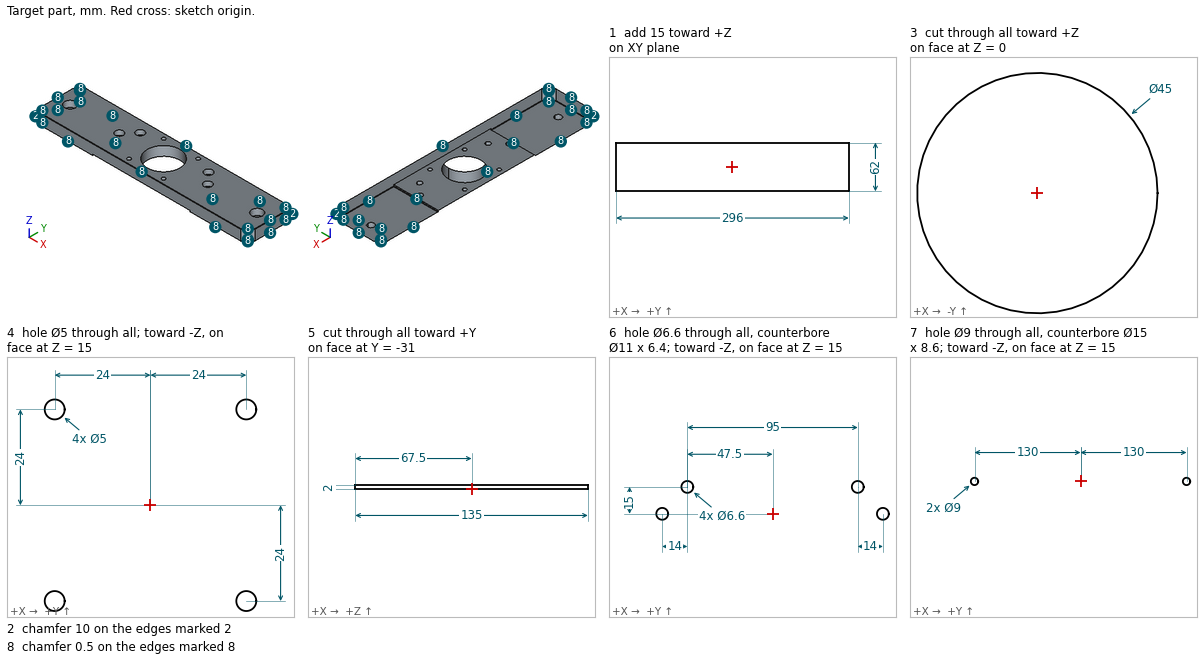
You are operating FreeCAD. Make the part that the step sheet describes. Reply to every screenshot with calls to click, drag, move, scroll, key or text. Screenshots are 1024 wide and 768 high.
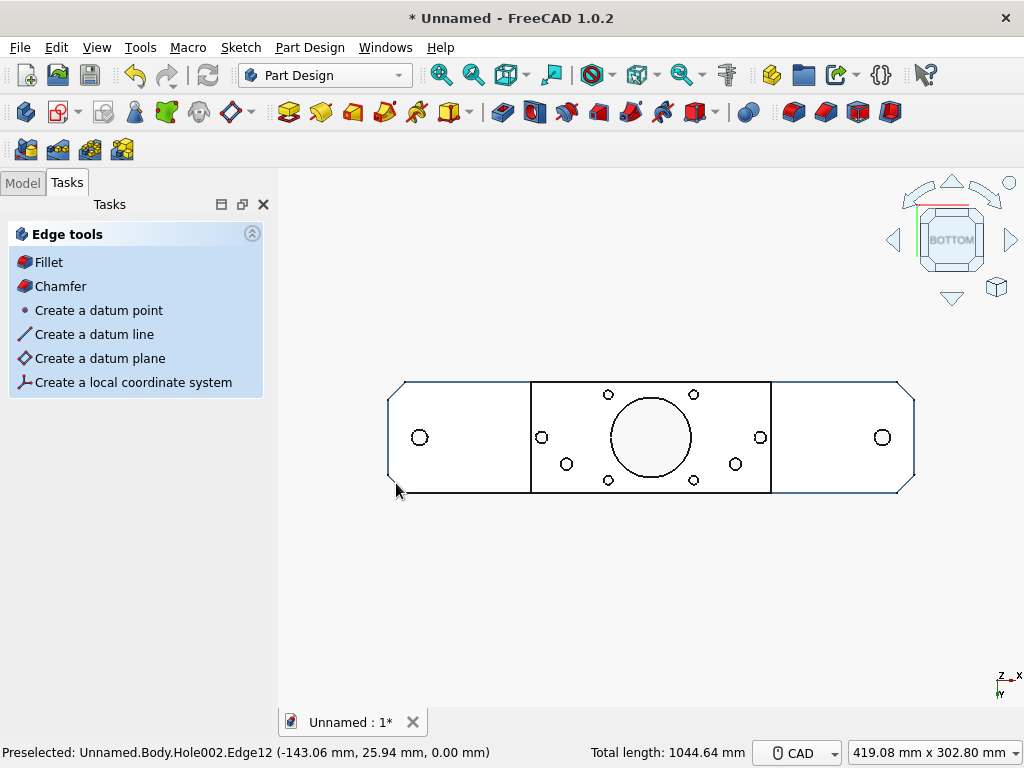
click(468, 492, ctrl)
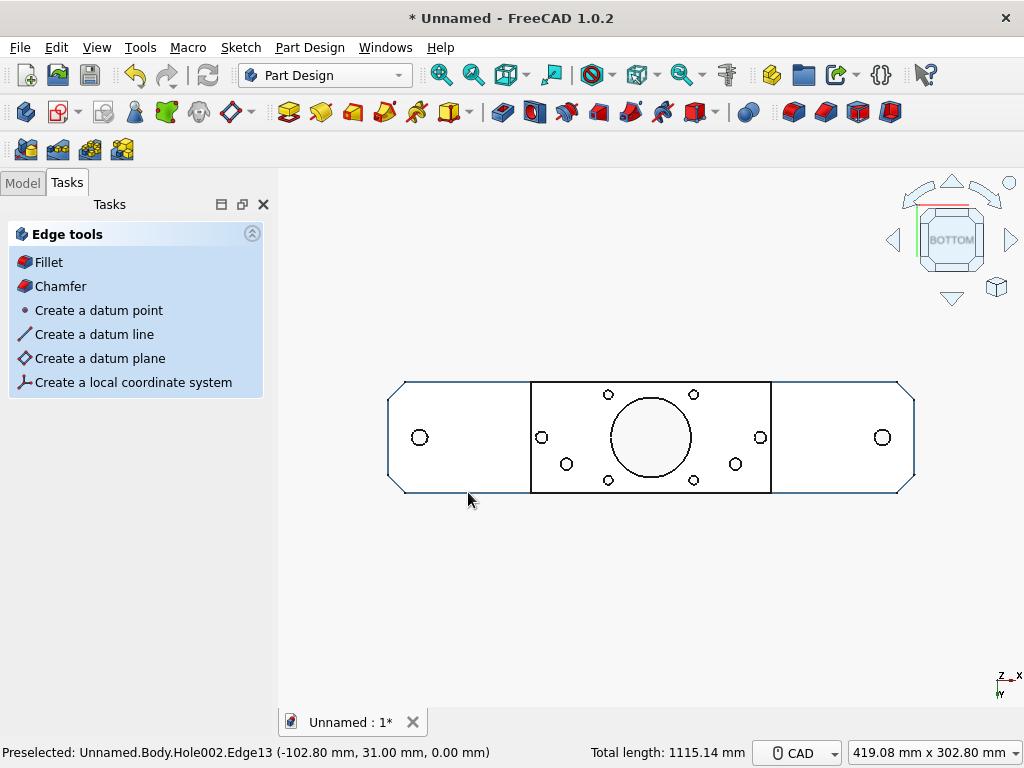
click(771, 436, ctrl)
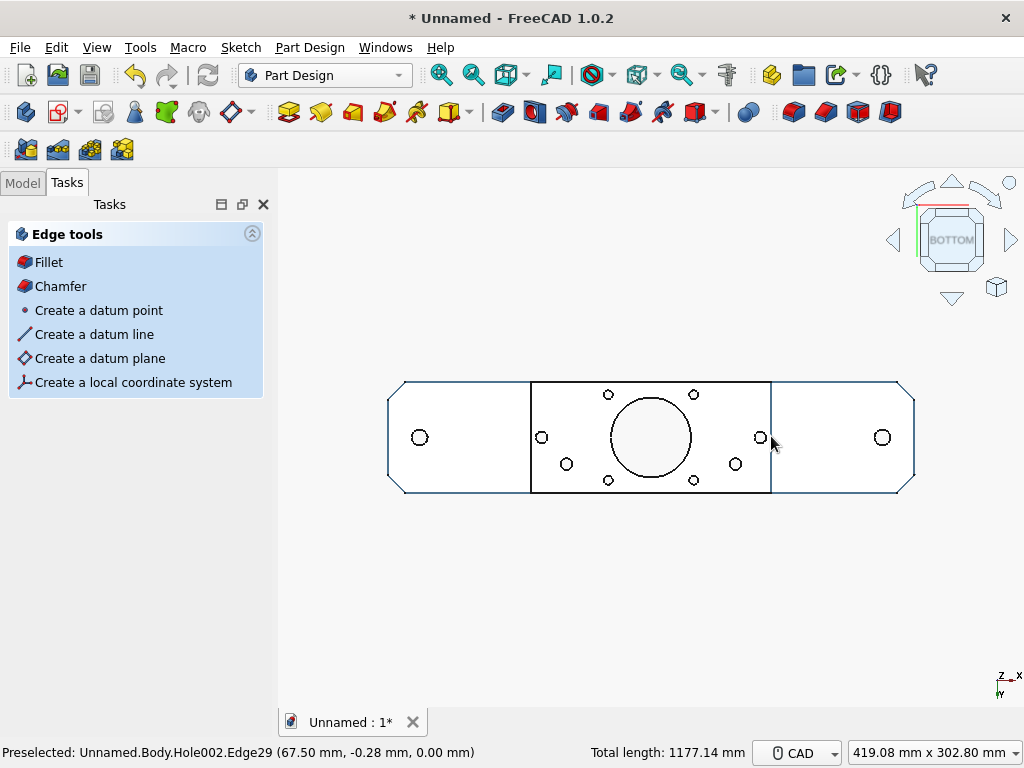
click(531, 436, ctrl)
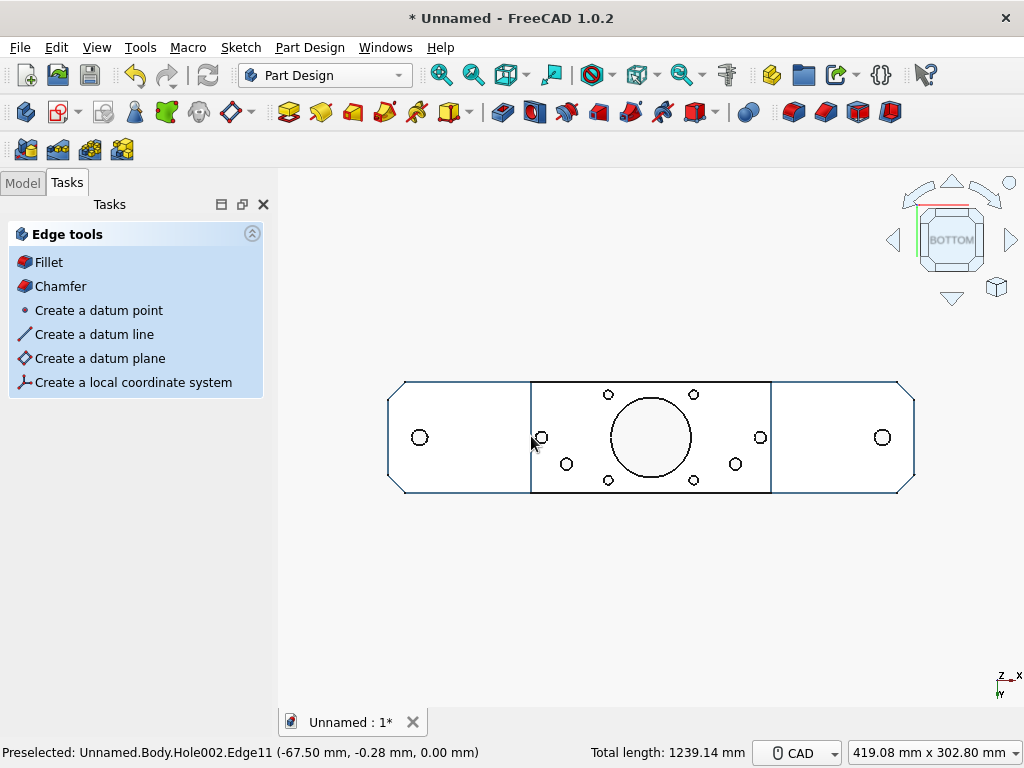
click(826, 112)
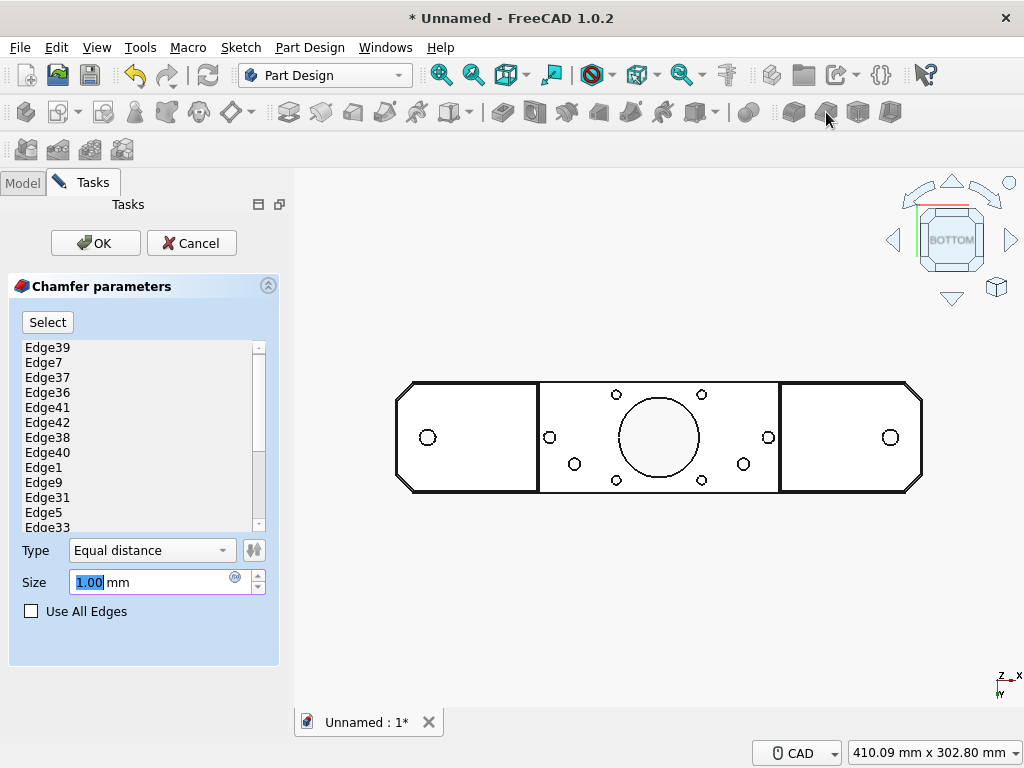
text(0.5)
key(Tab)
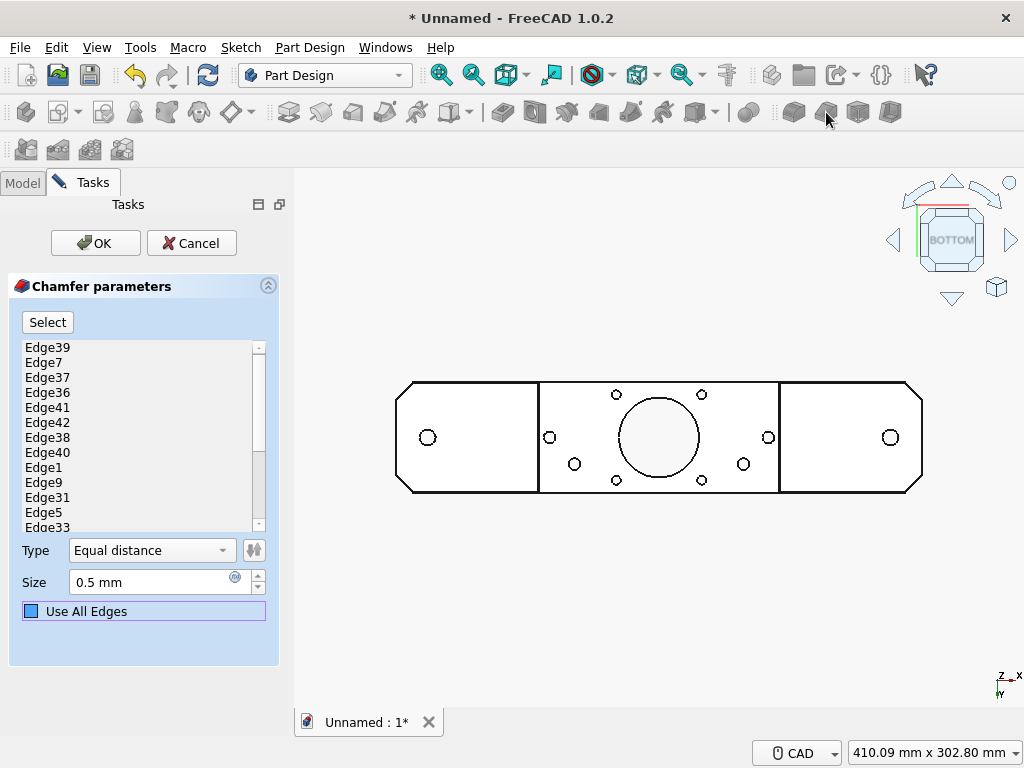
click(96, 243)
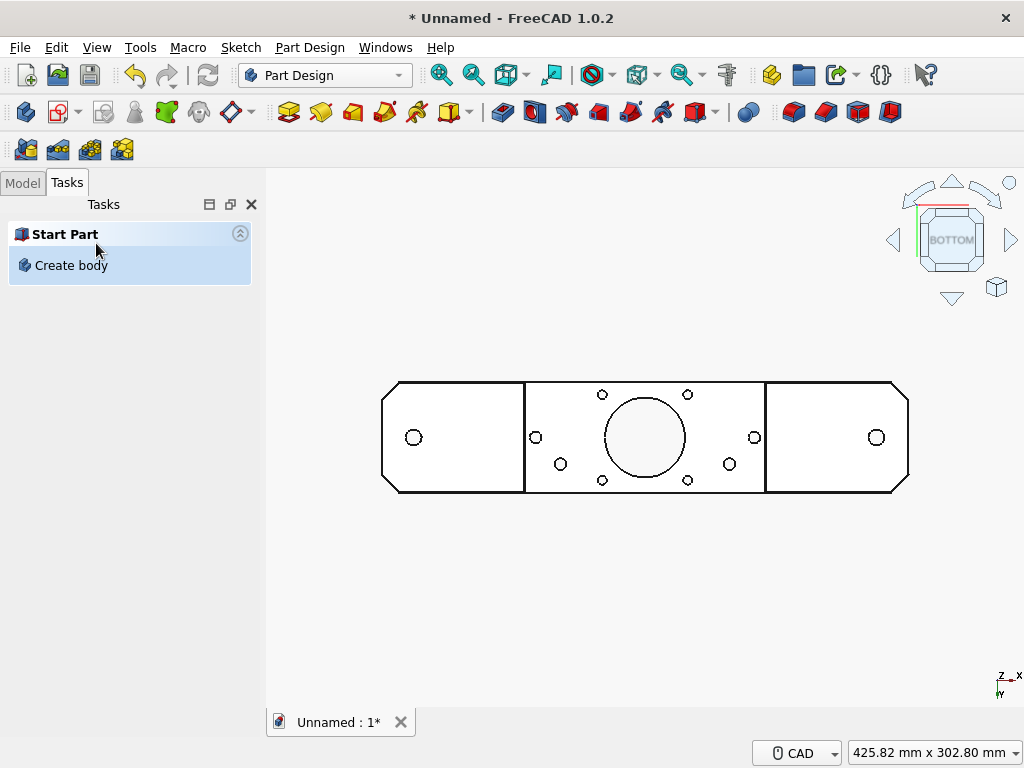
key(0)